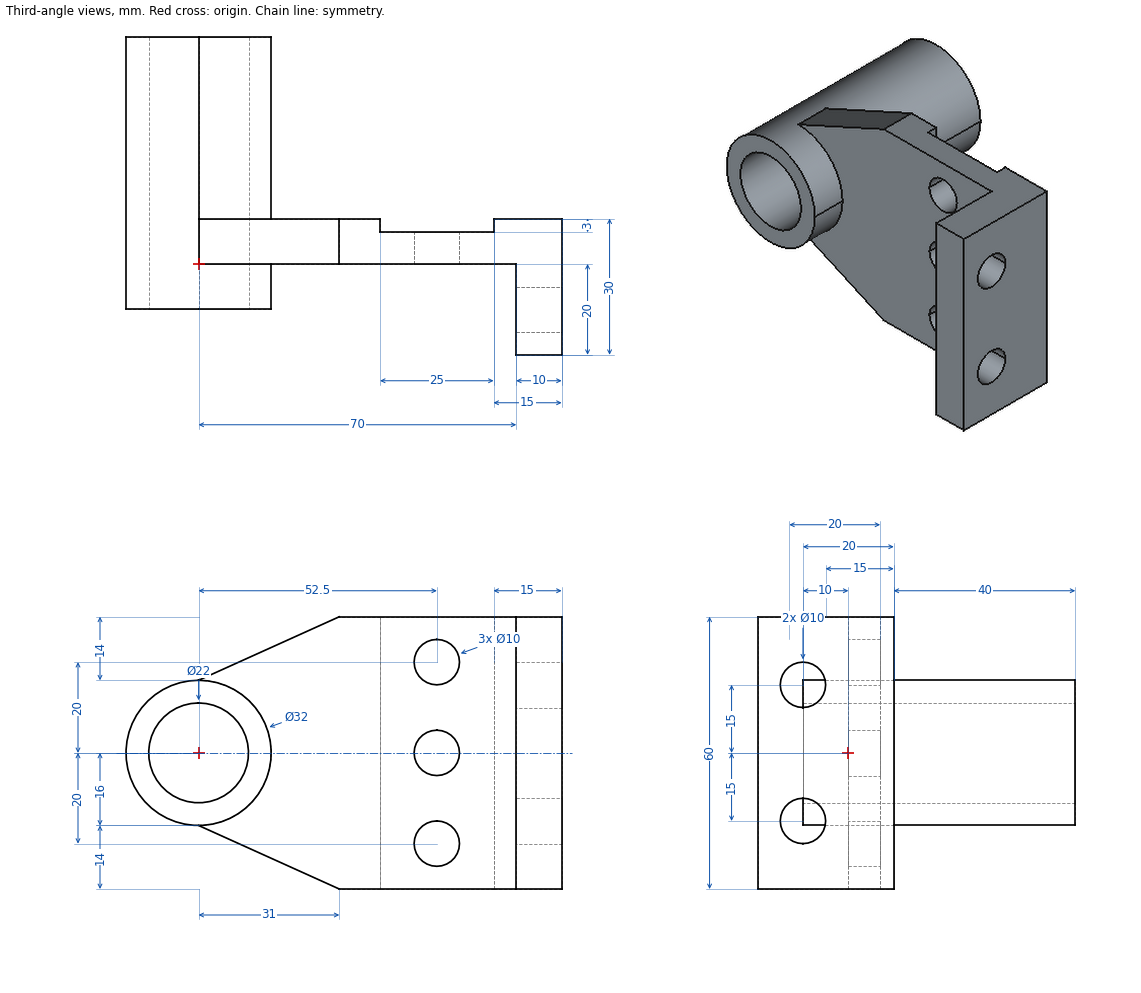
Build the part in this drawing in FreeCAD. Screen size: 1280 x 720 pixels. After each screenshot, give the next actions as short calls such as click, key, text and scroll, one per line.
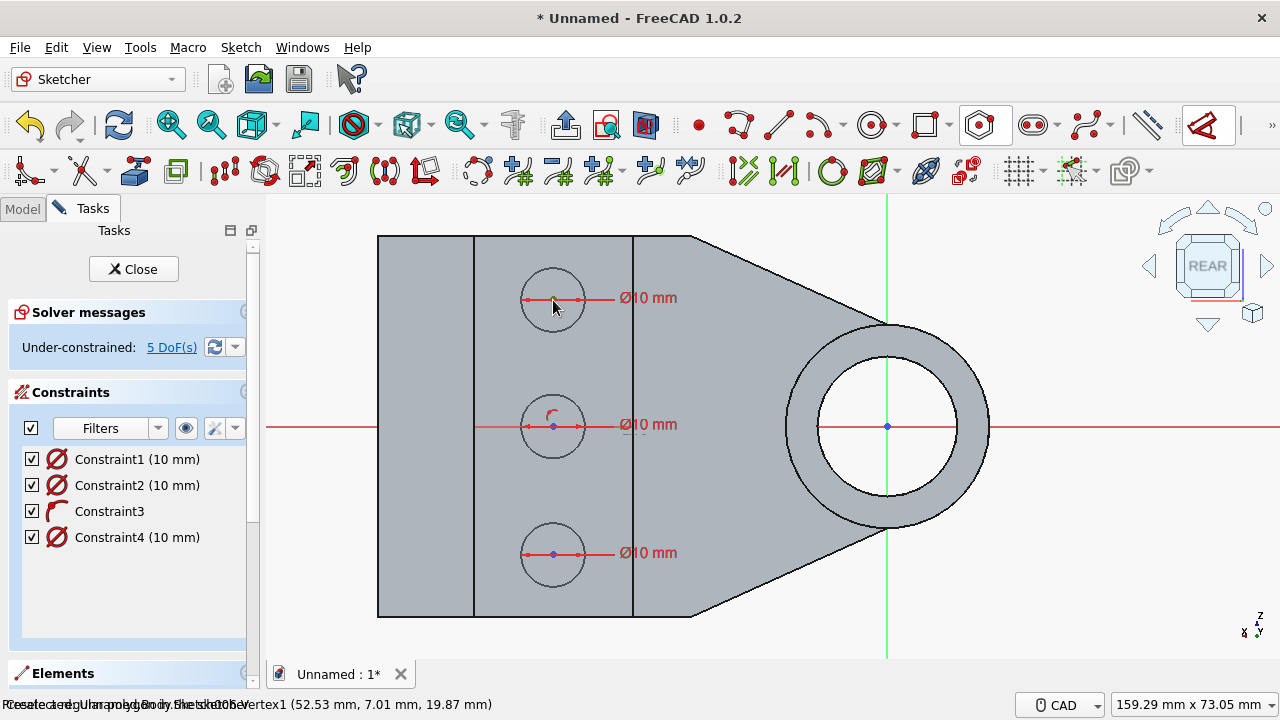
click(553, 426)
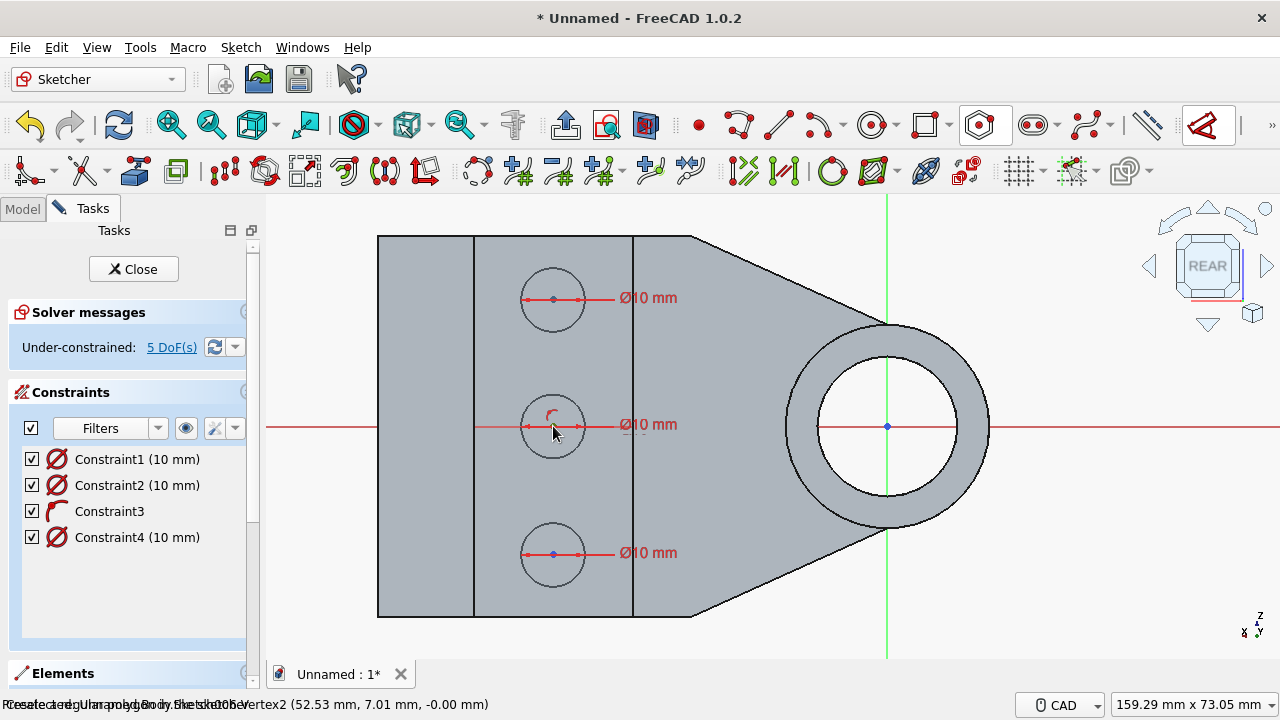
key(v)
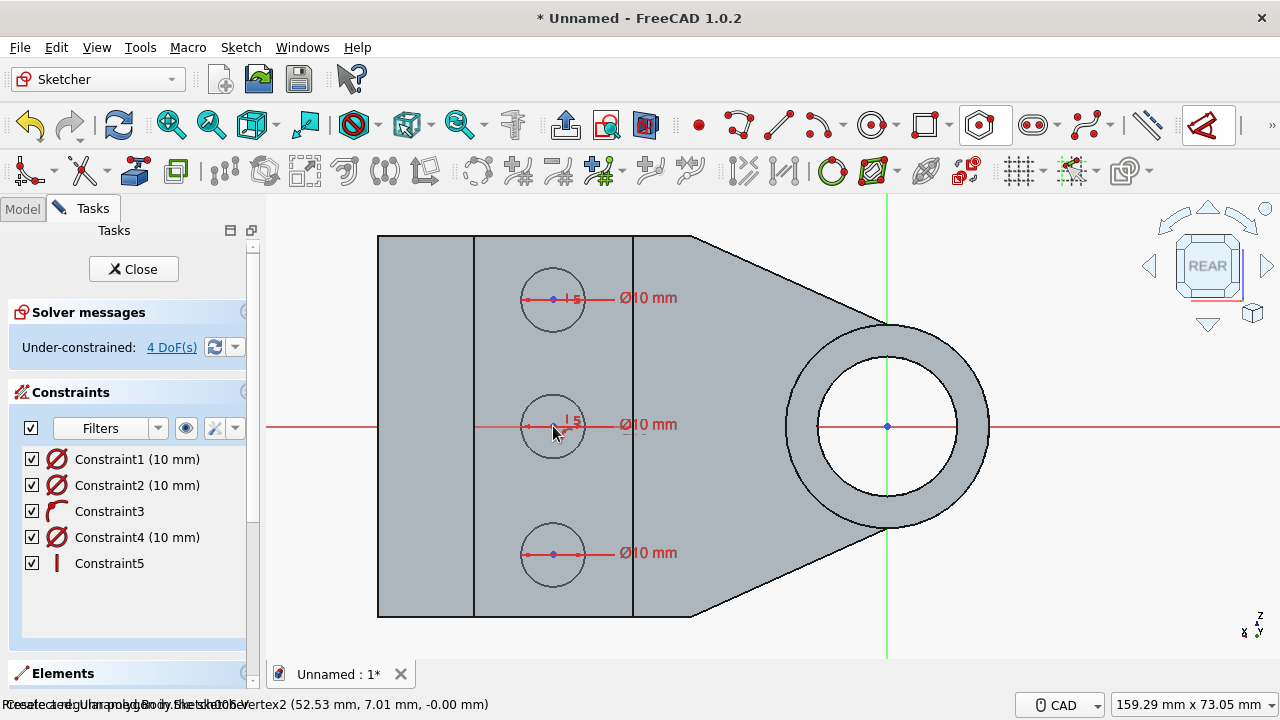
click(553, 426)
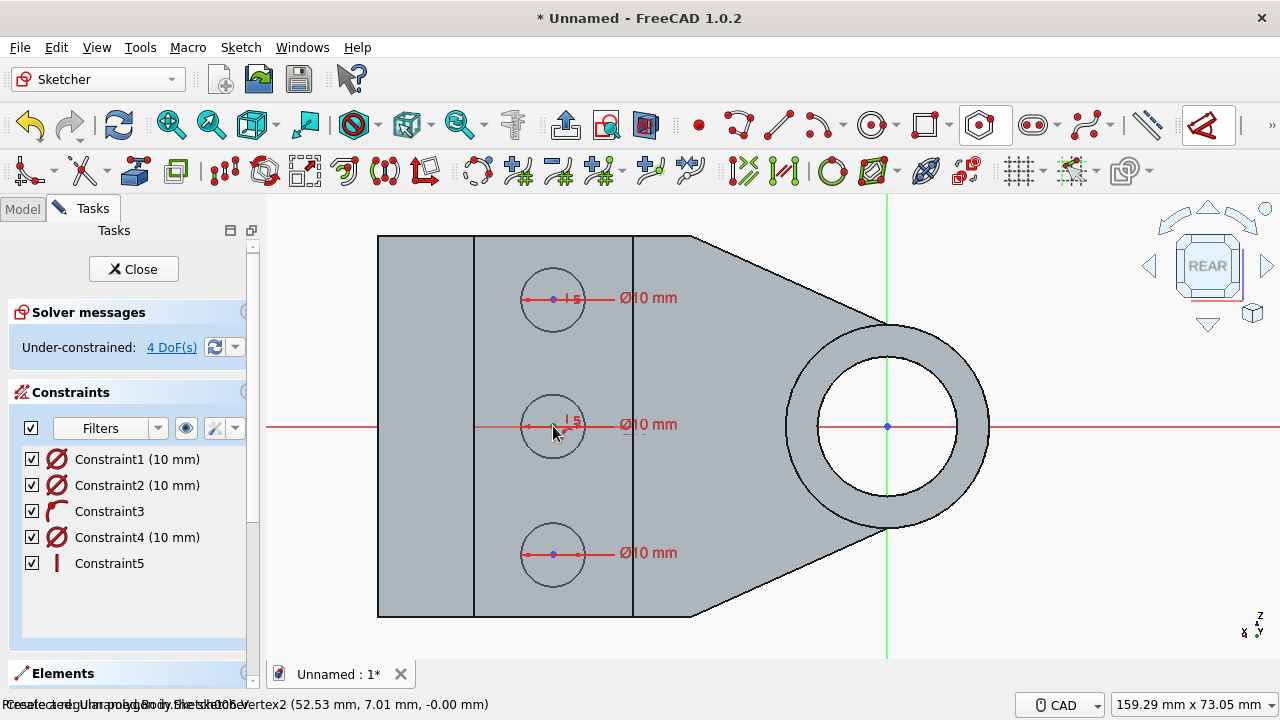
click(553, 555)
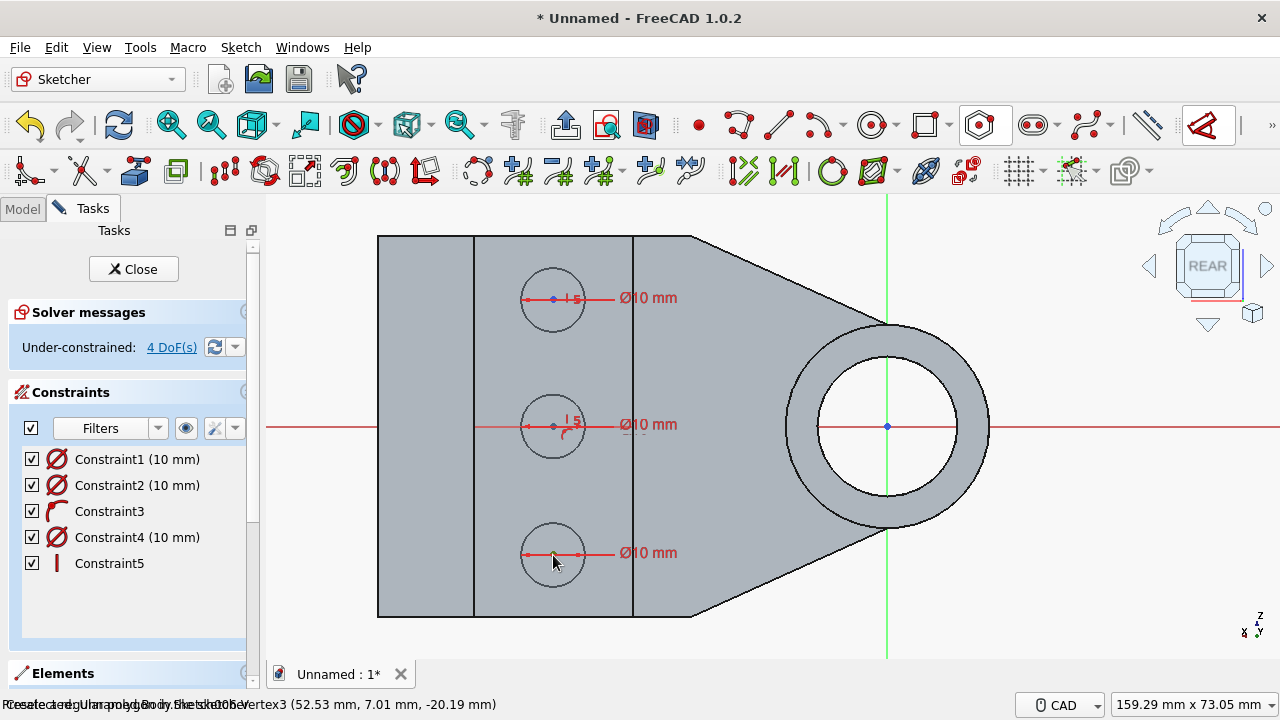
key(v)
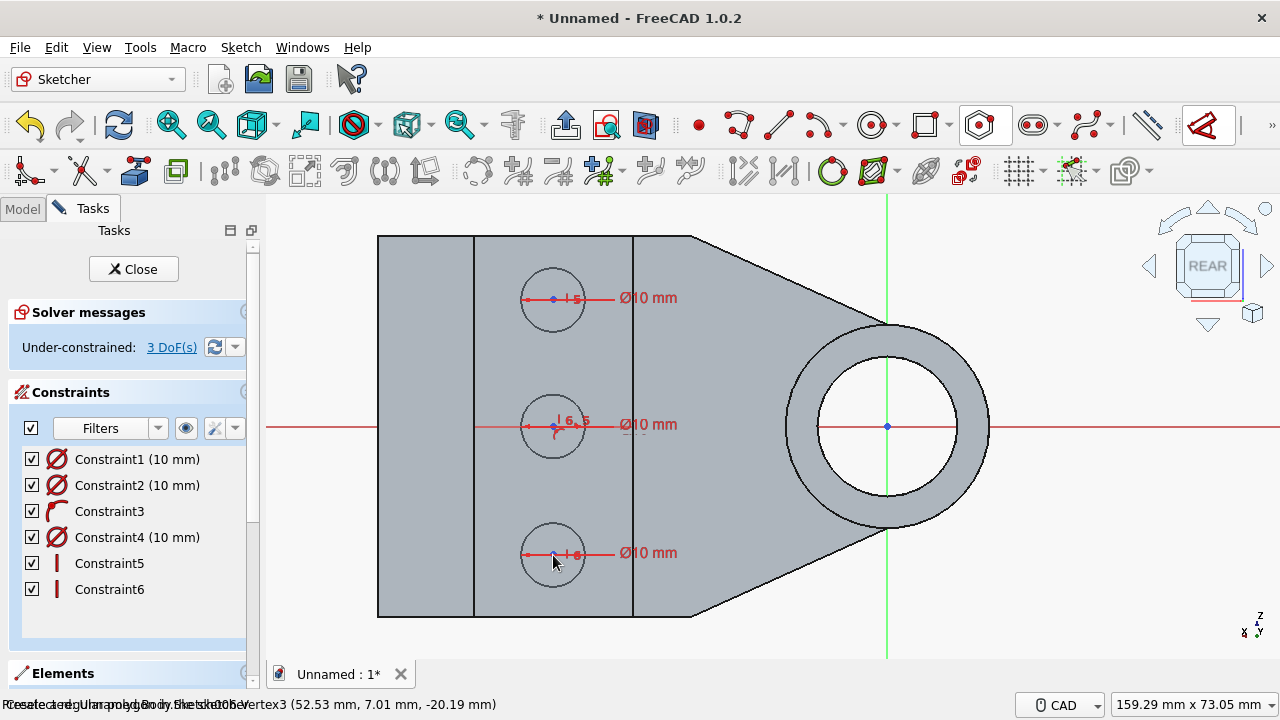
click(553, 300)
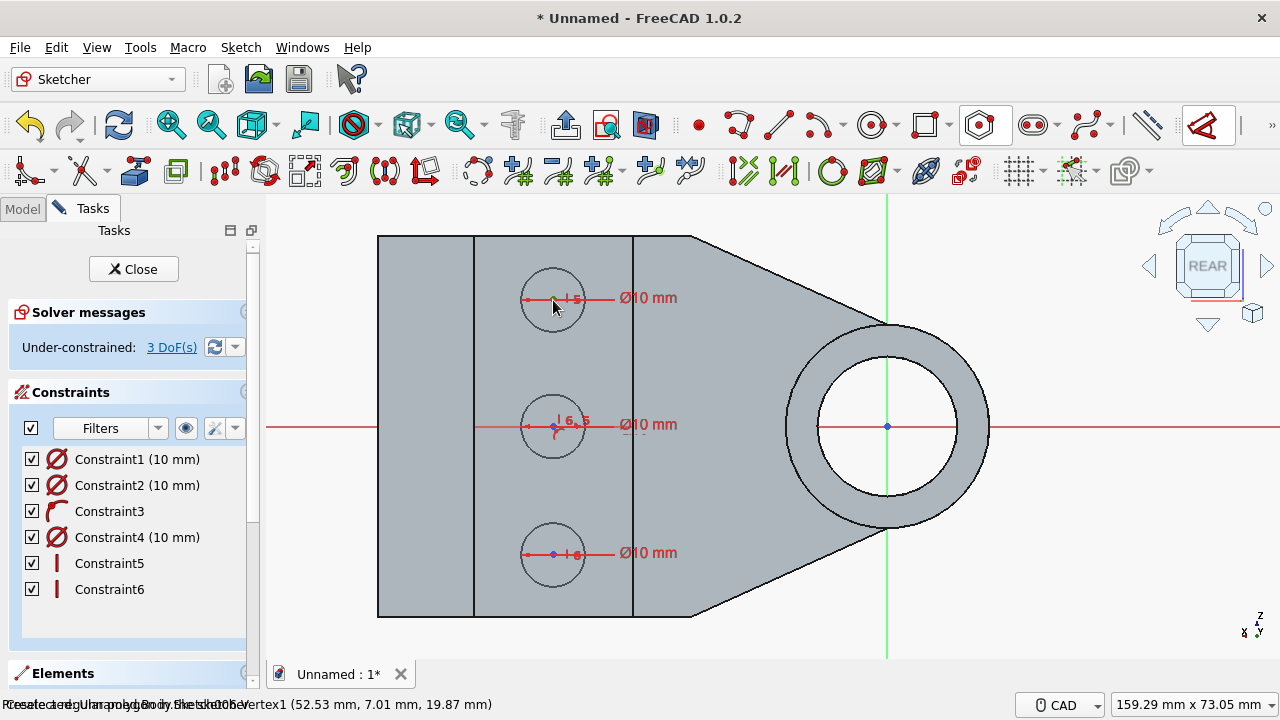
click(1230, 126)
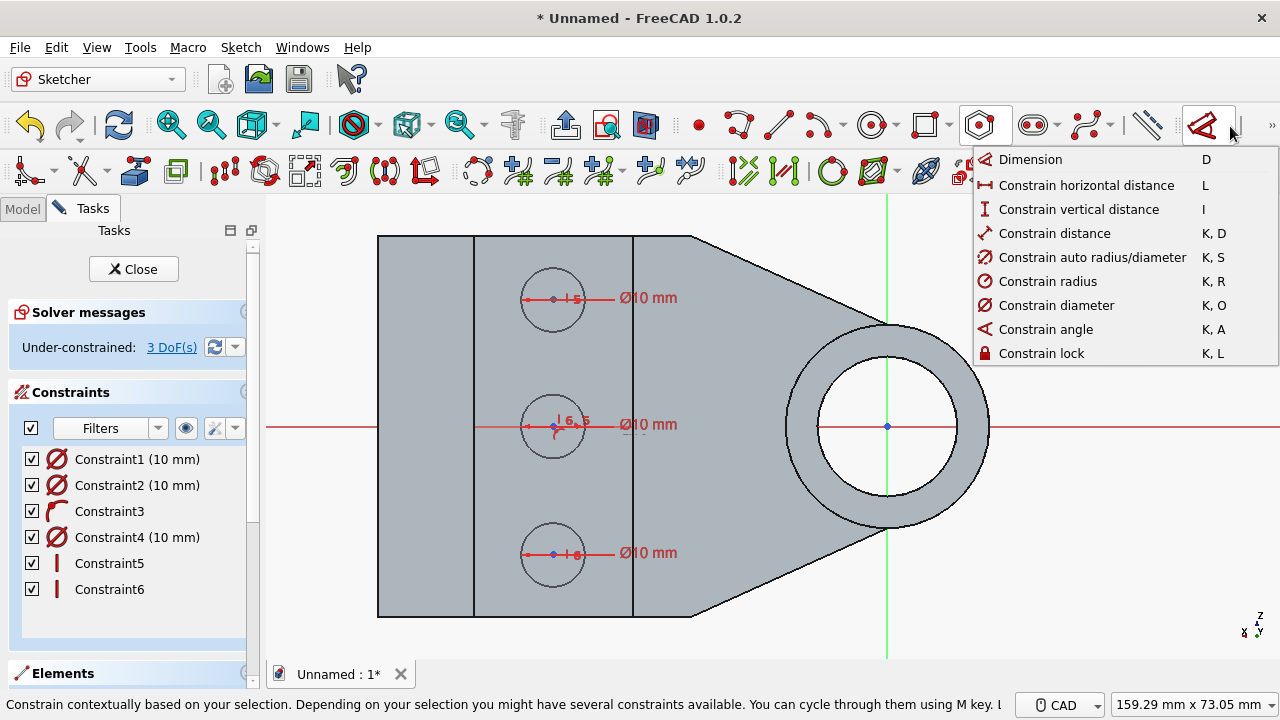
click(1126, 209)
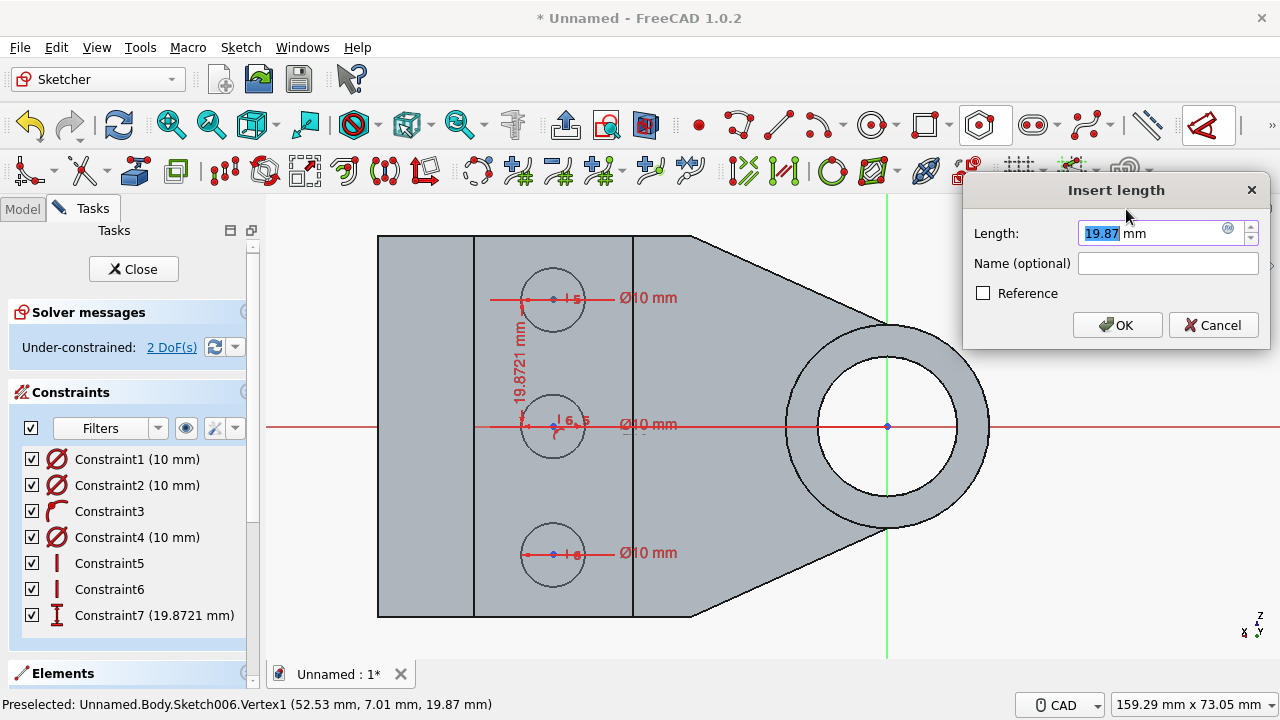
text(20)
key(Return)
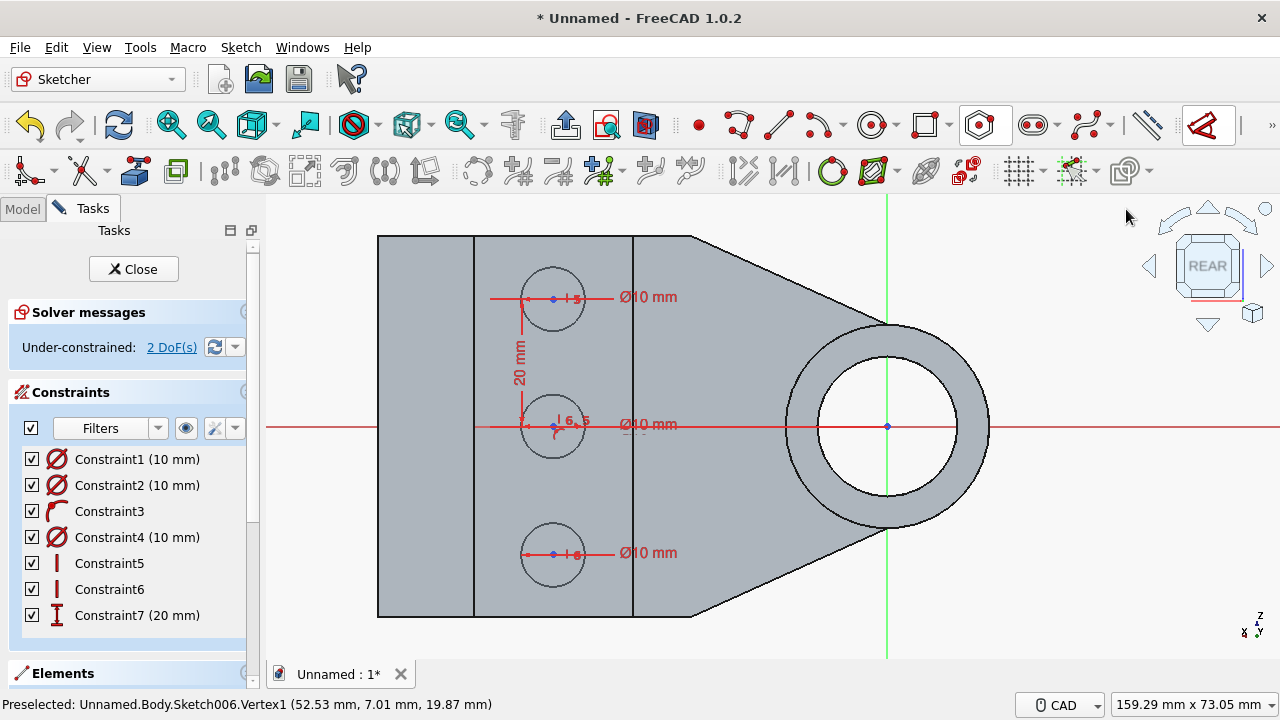
click(553, 555)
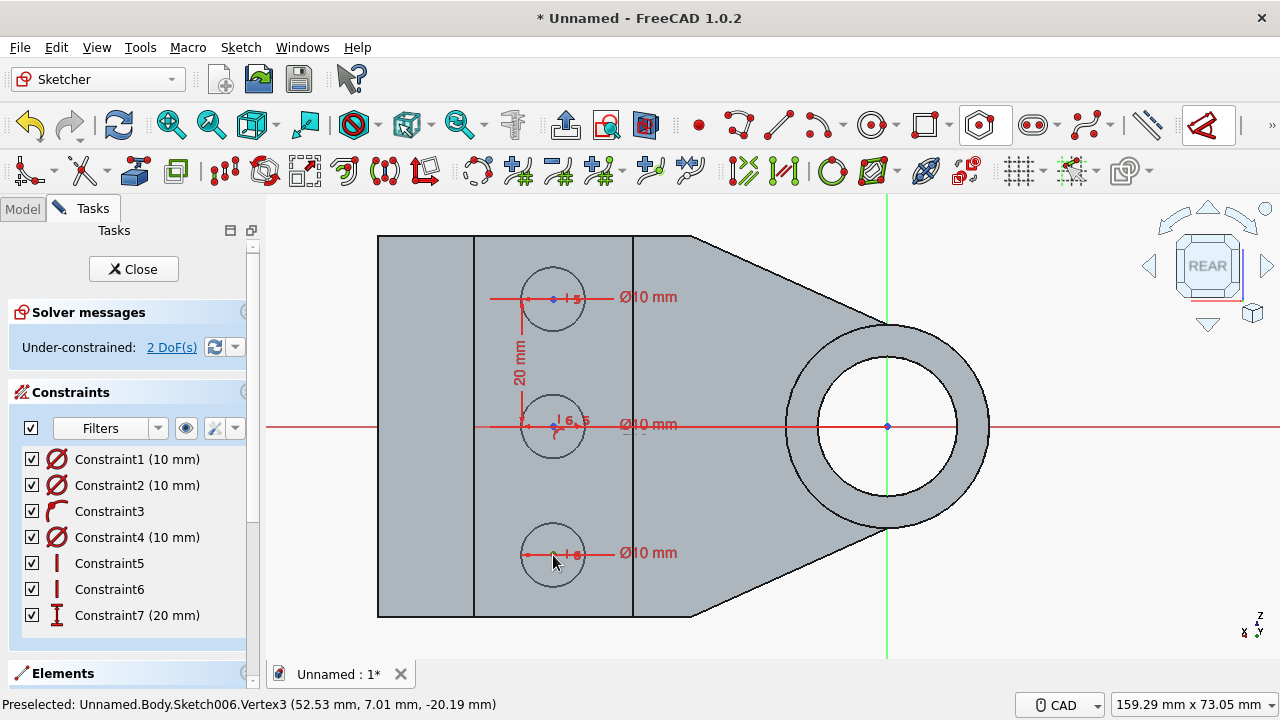
click(1230, 126)